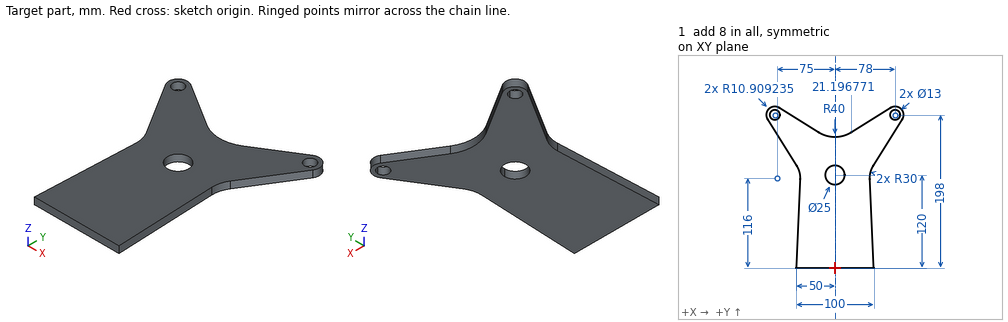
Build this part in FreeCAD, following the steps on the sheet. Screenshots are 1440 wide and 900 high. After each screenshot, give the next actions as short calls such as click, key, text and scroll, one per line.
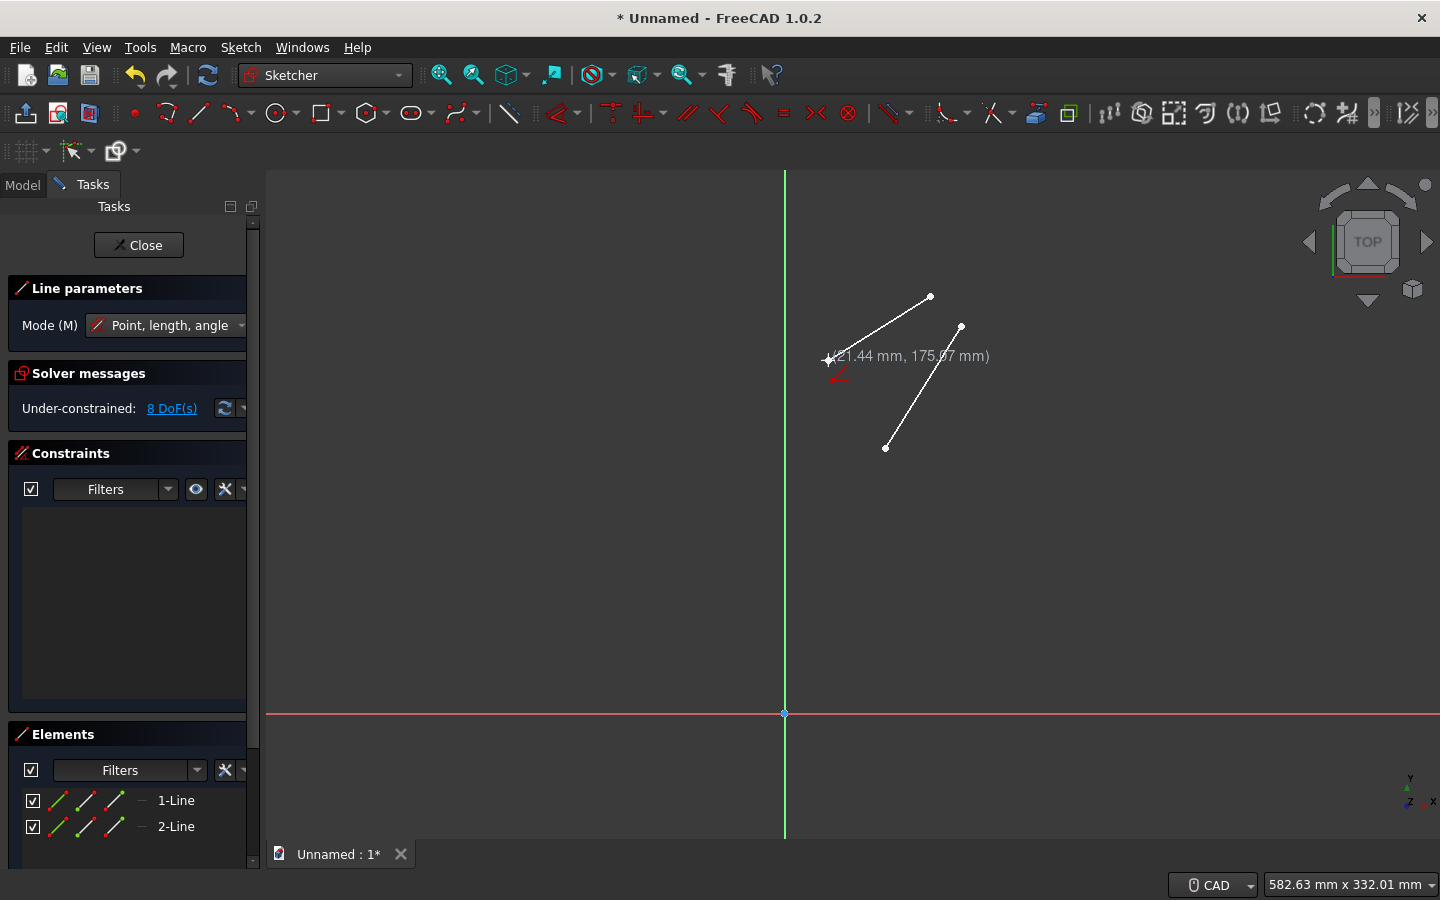
click(742, 360)
click(639, 296)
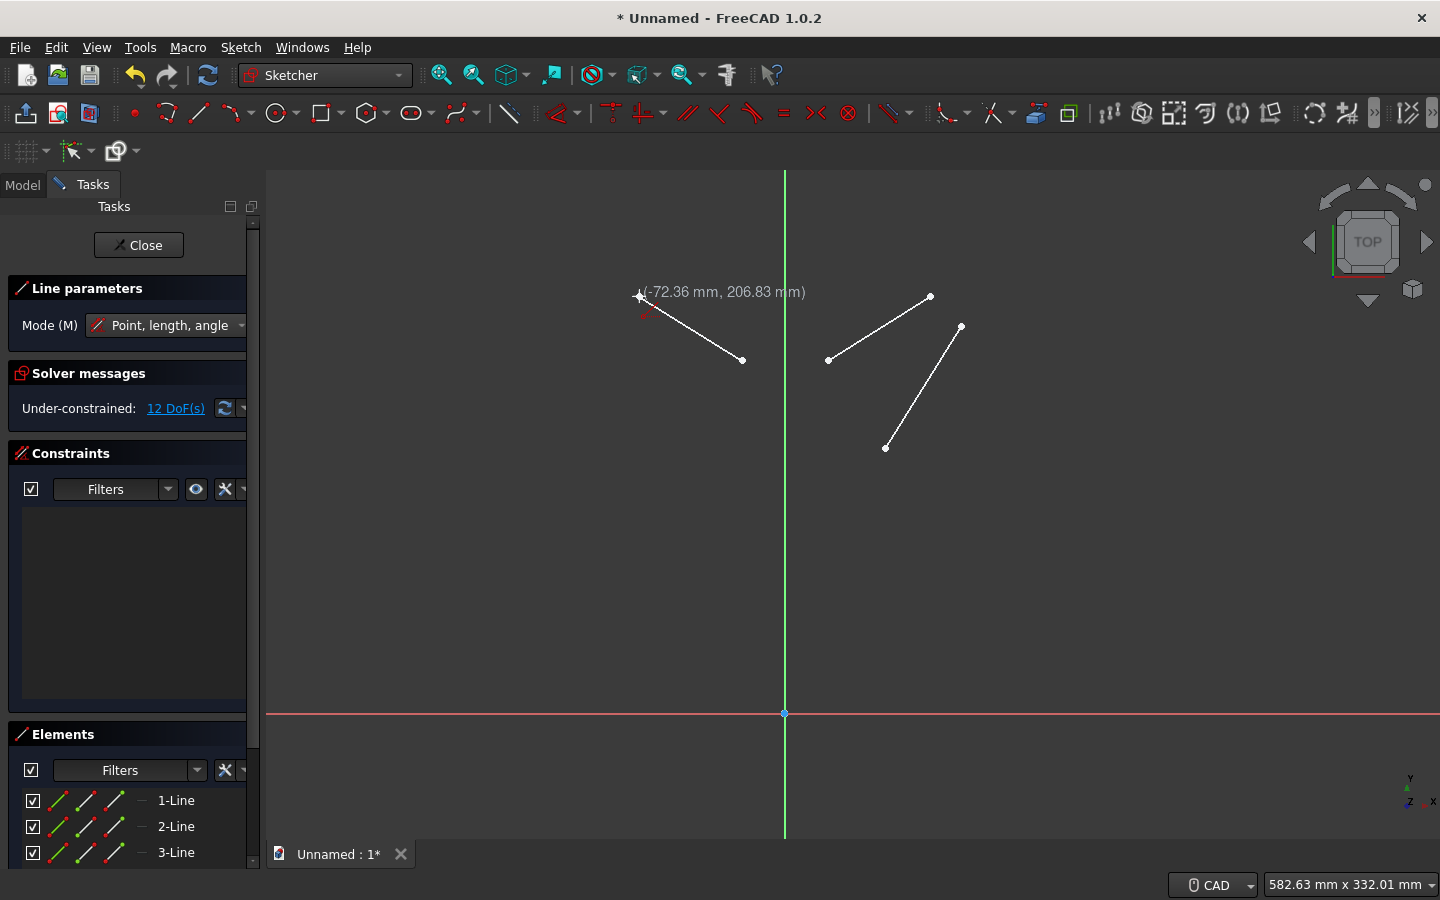
click(609, 326)
click(685, 448)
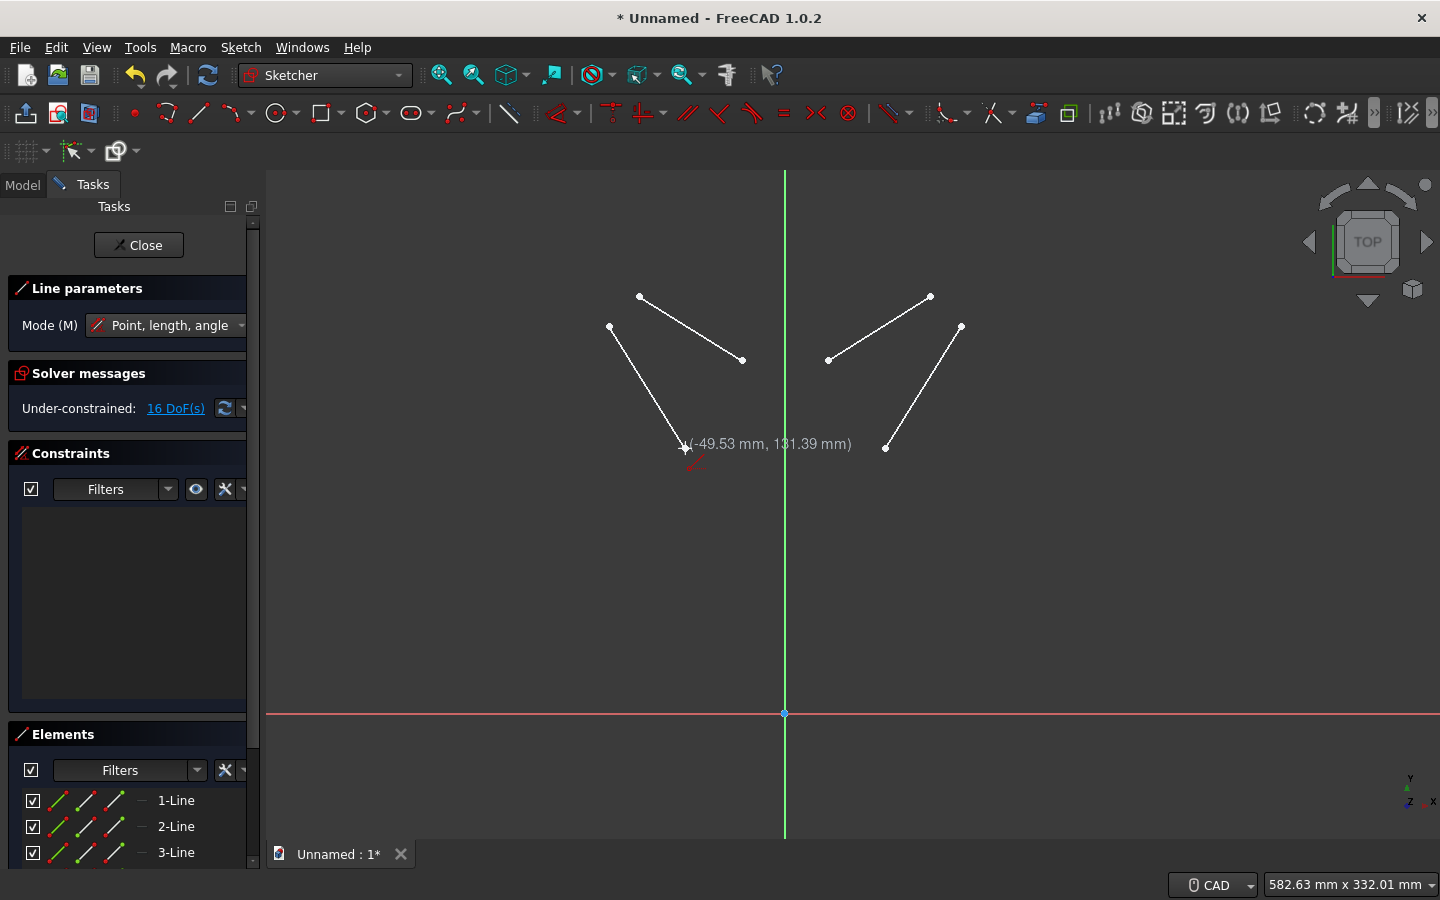
click(168, 114)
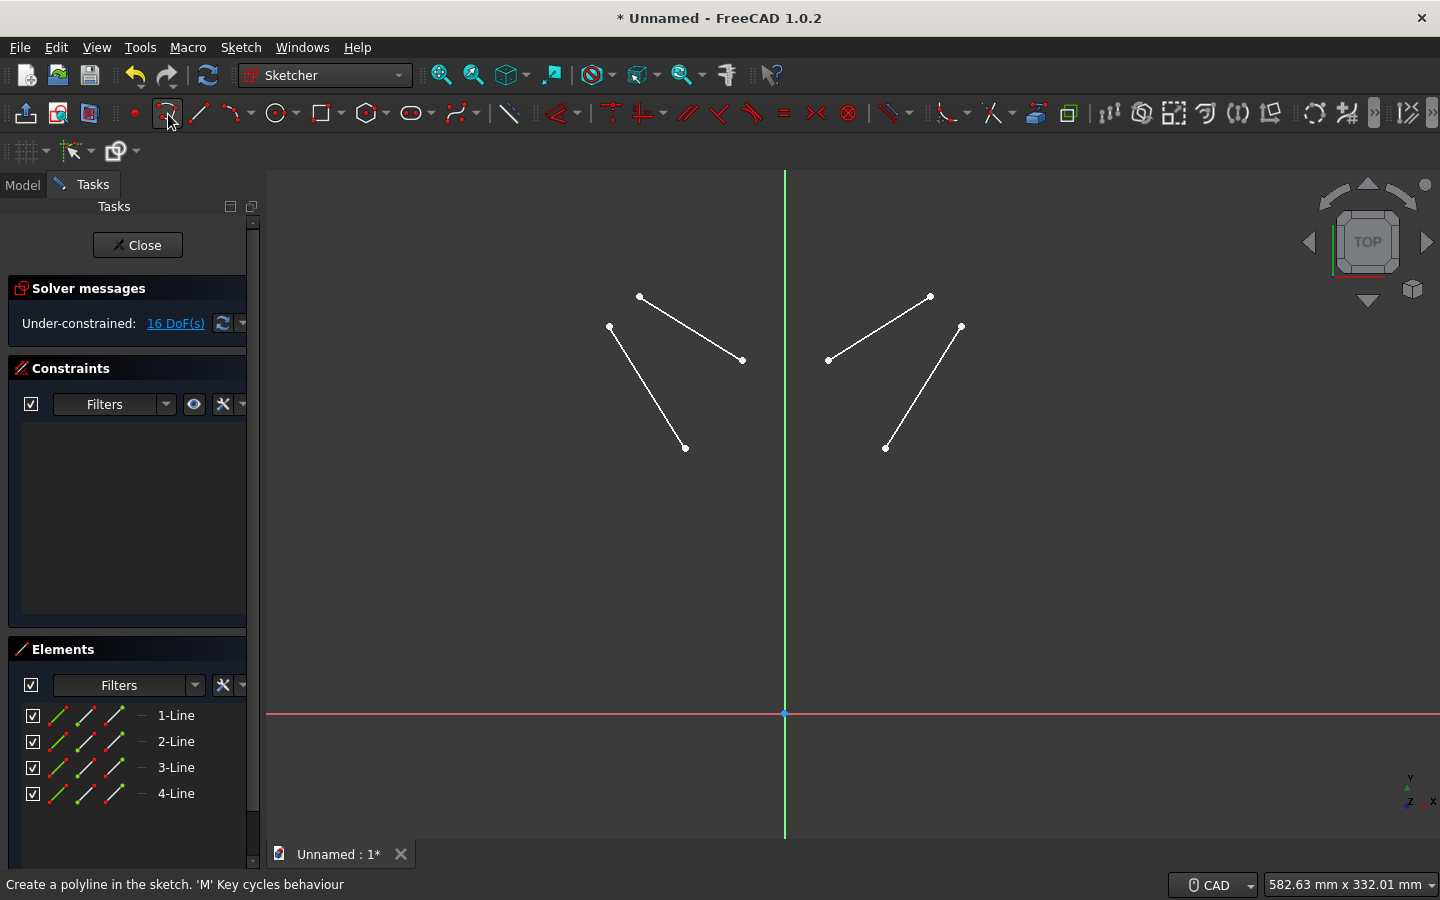
click(694, 483)
click(682, 714)
click(886, 705)
click(874, 483)
right_click(874, 483)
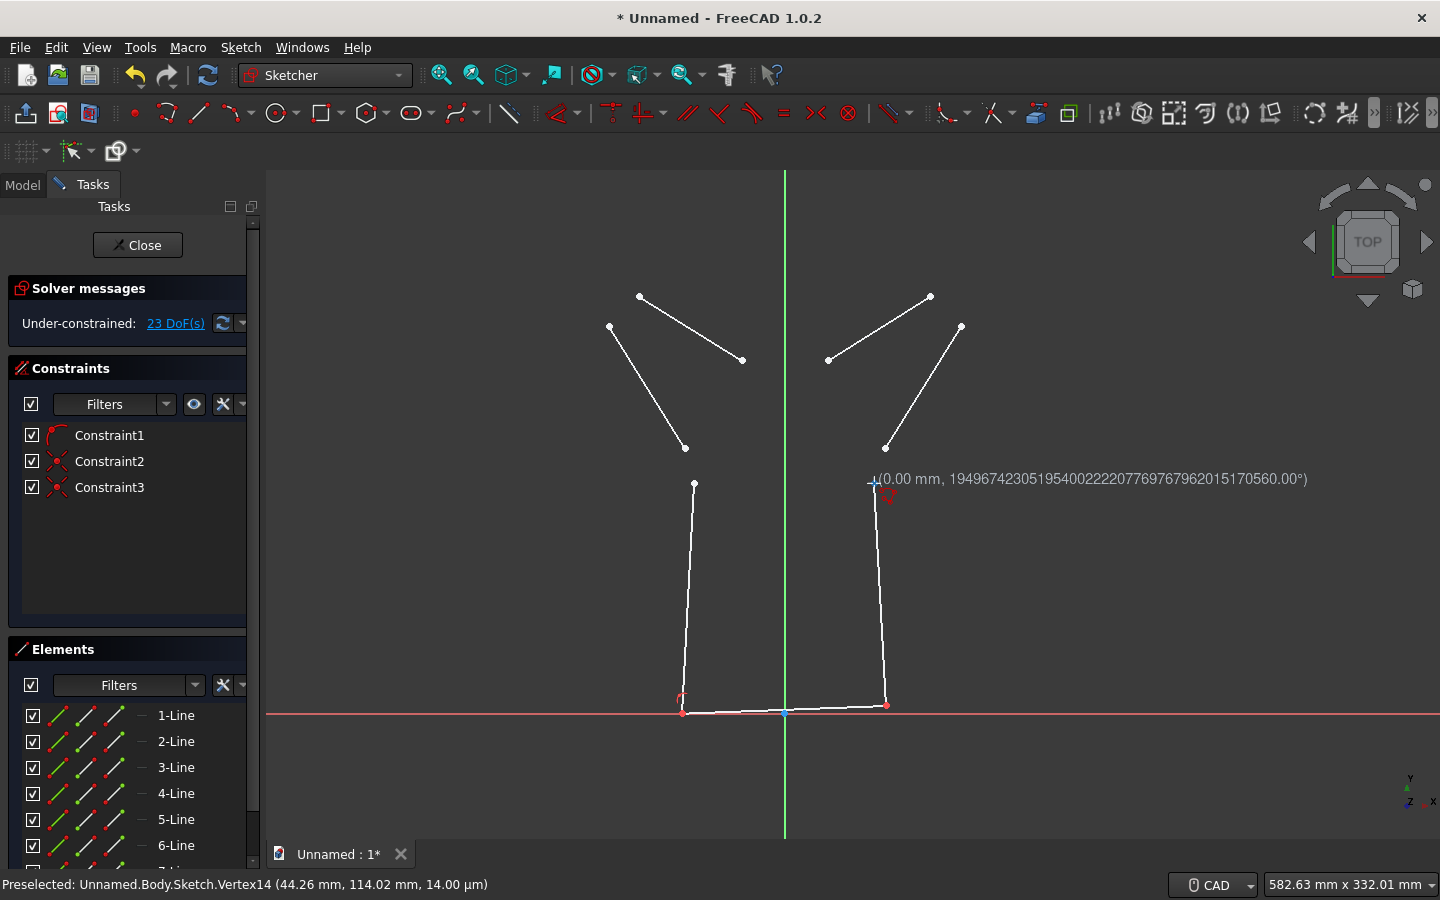
key(g)
key(3)
key(a)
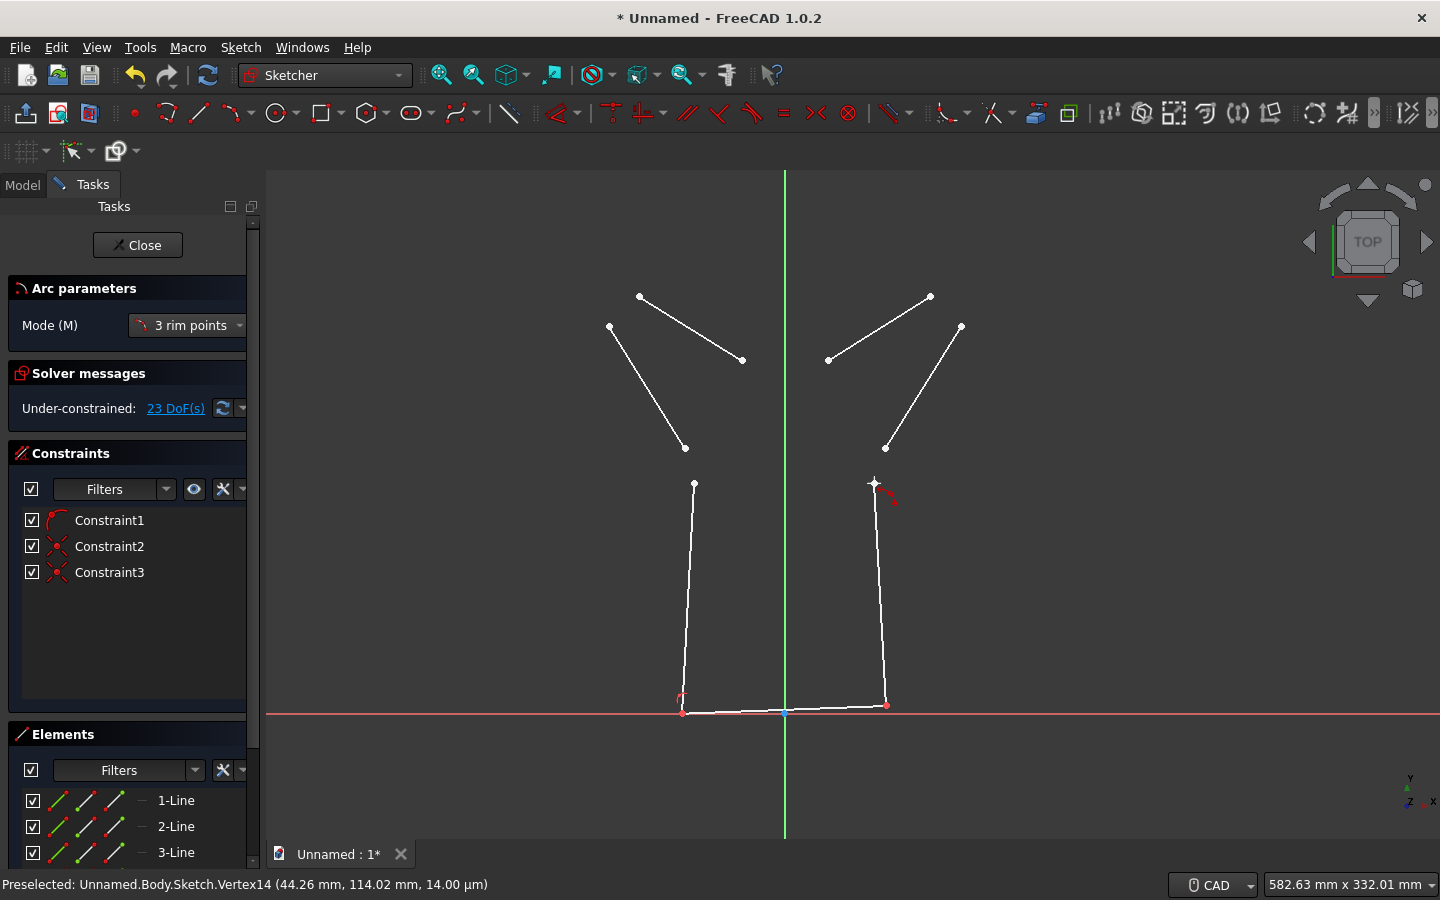
click(961, 327)
click(930, 297)
click(958, 299)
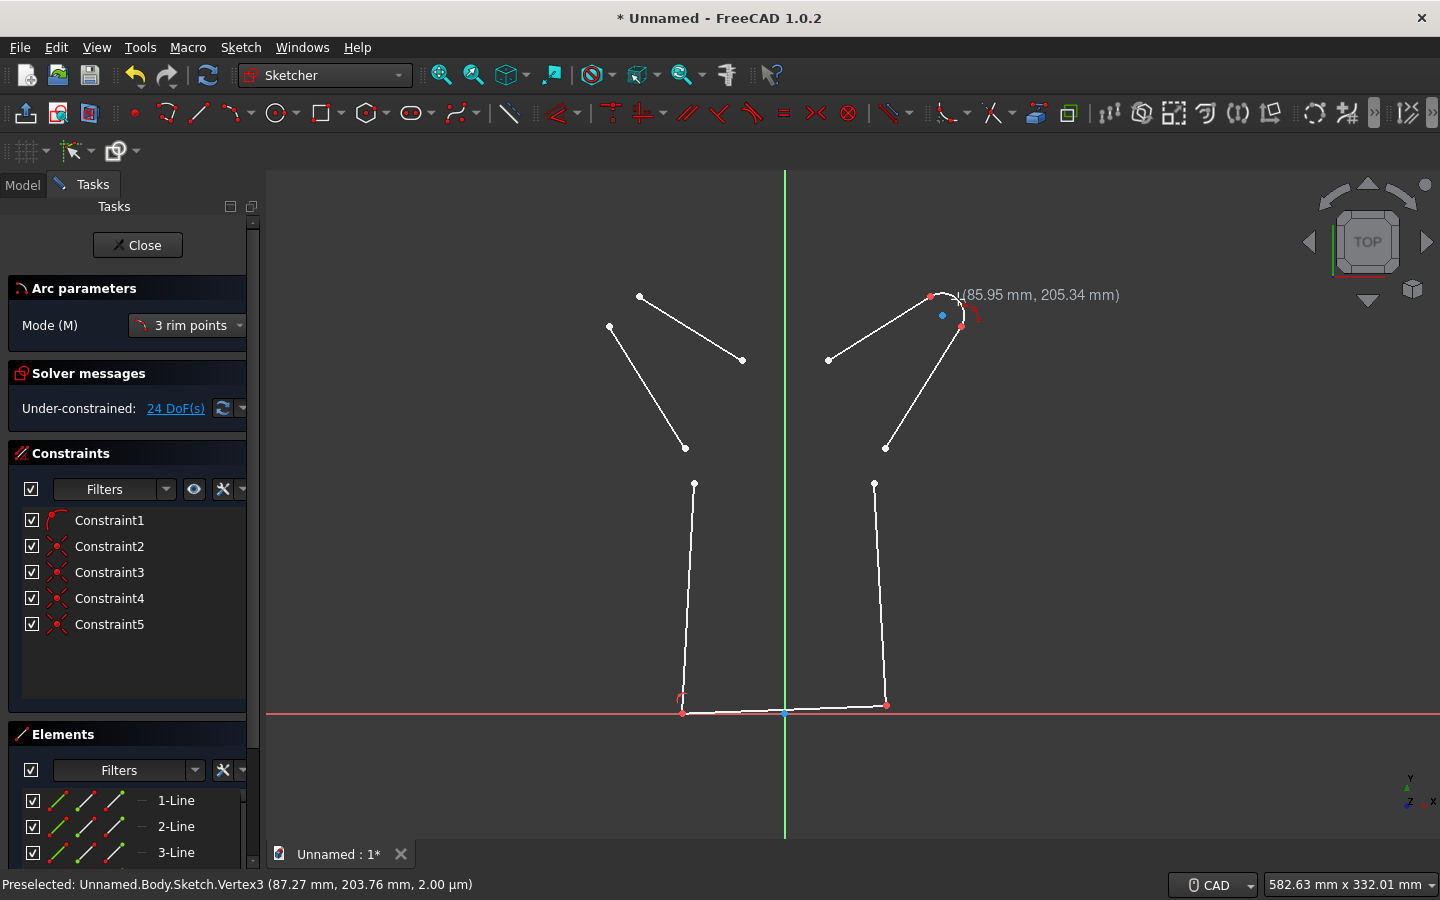
click(828, 361)
click(742, 361)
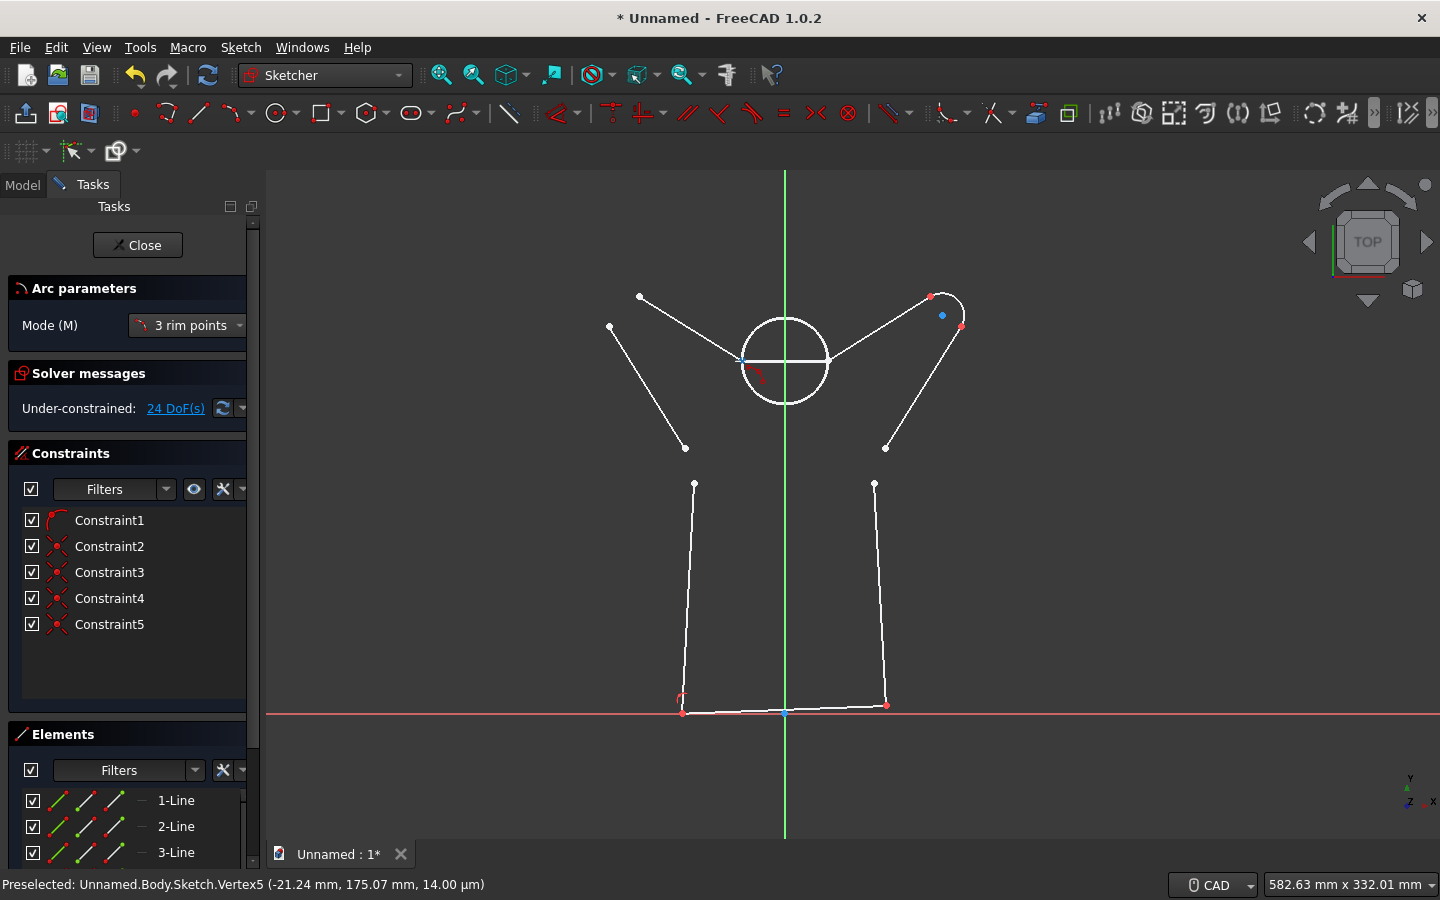
scroll(767, 371, up, 3)